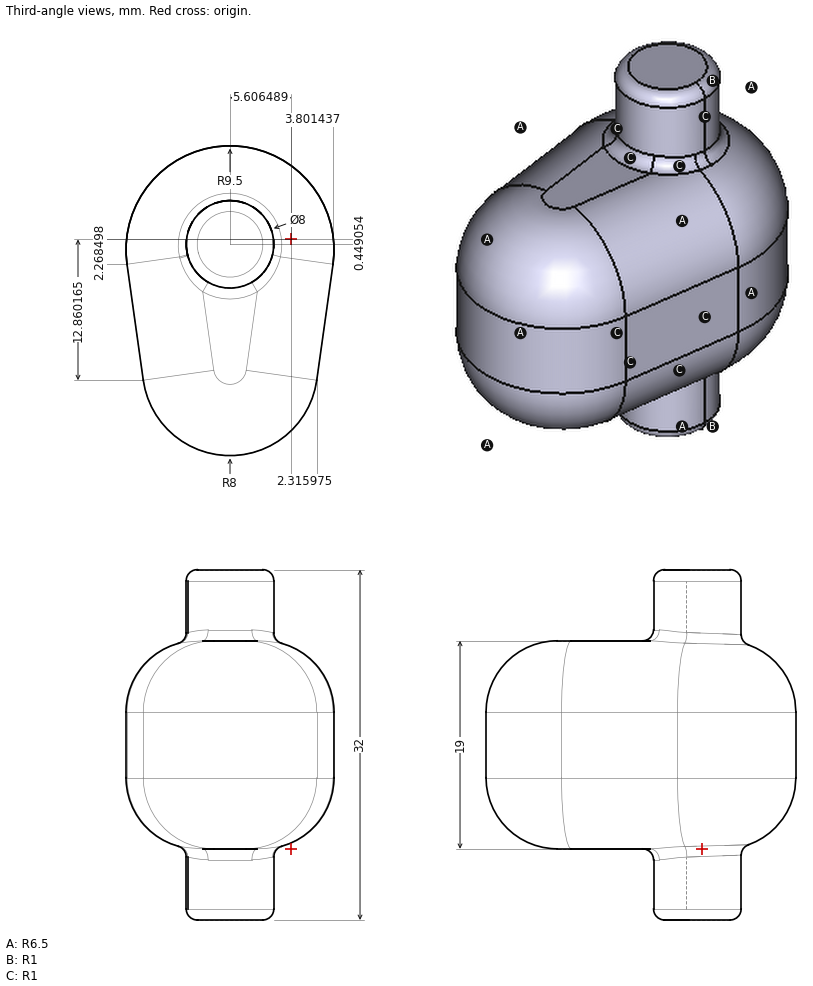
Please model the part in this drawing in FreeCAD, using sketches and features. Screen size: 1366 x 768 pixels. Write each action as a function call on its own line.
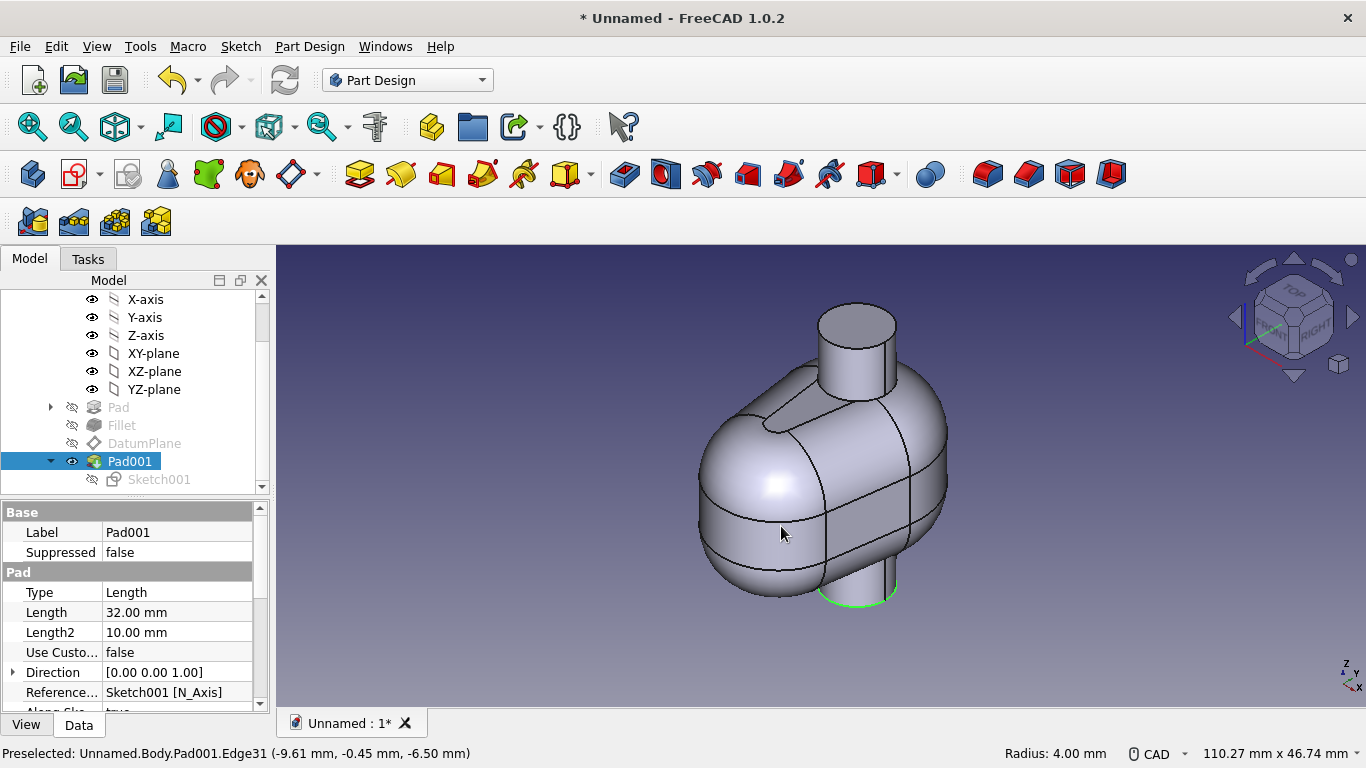
click(818, 321, ctrl)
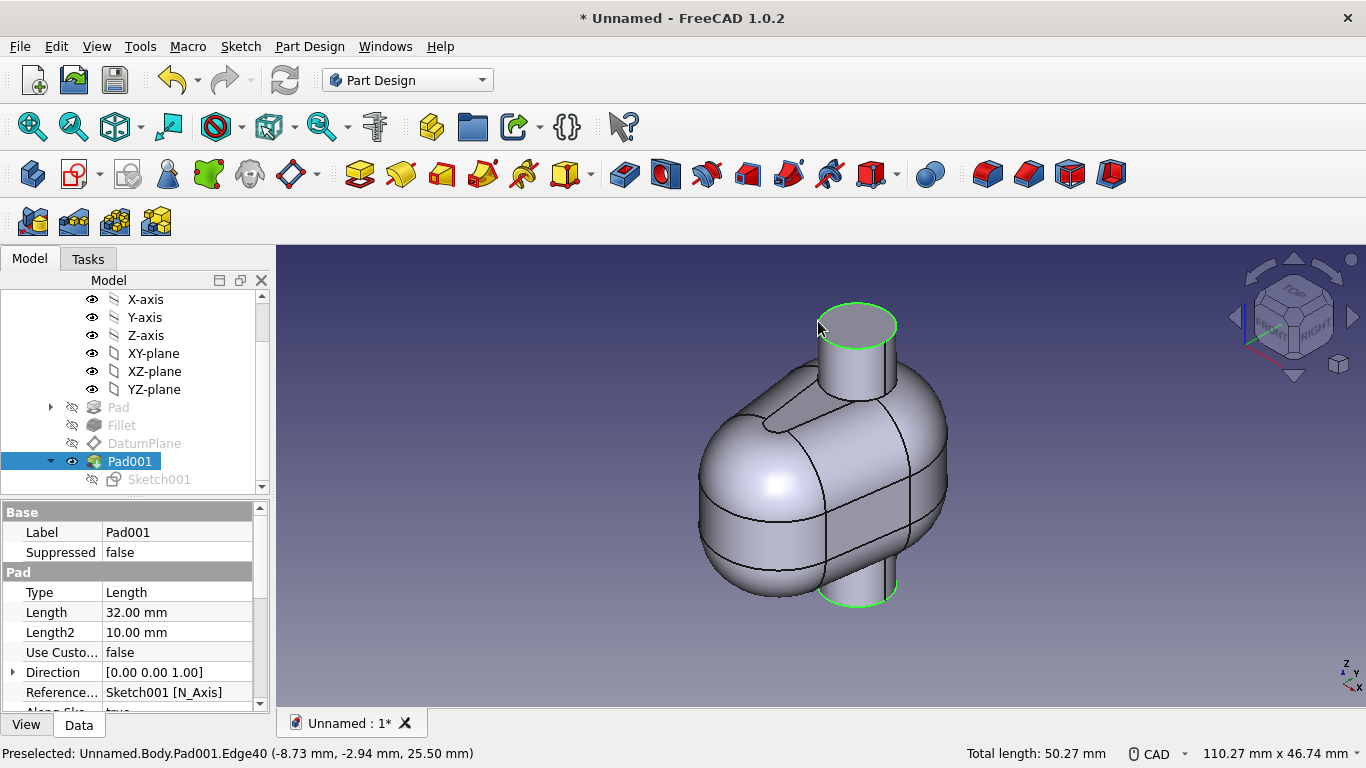
click(988, 174)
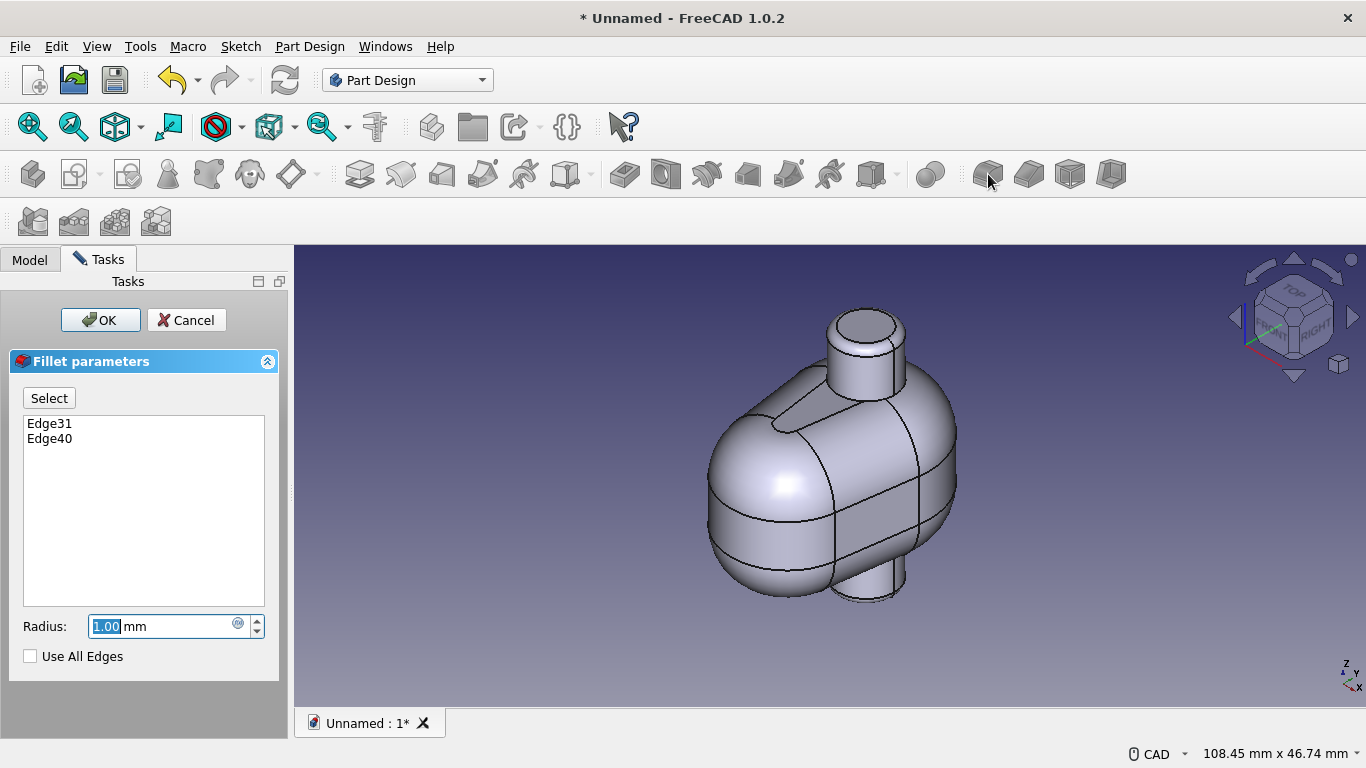
text(1)
key(Tab)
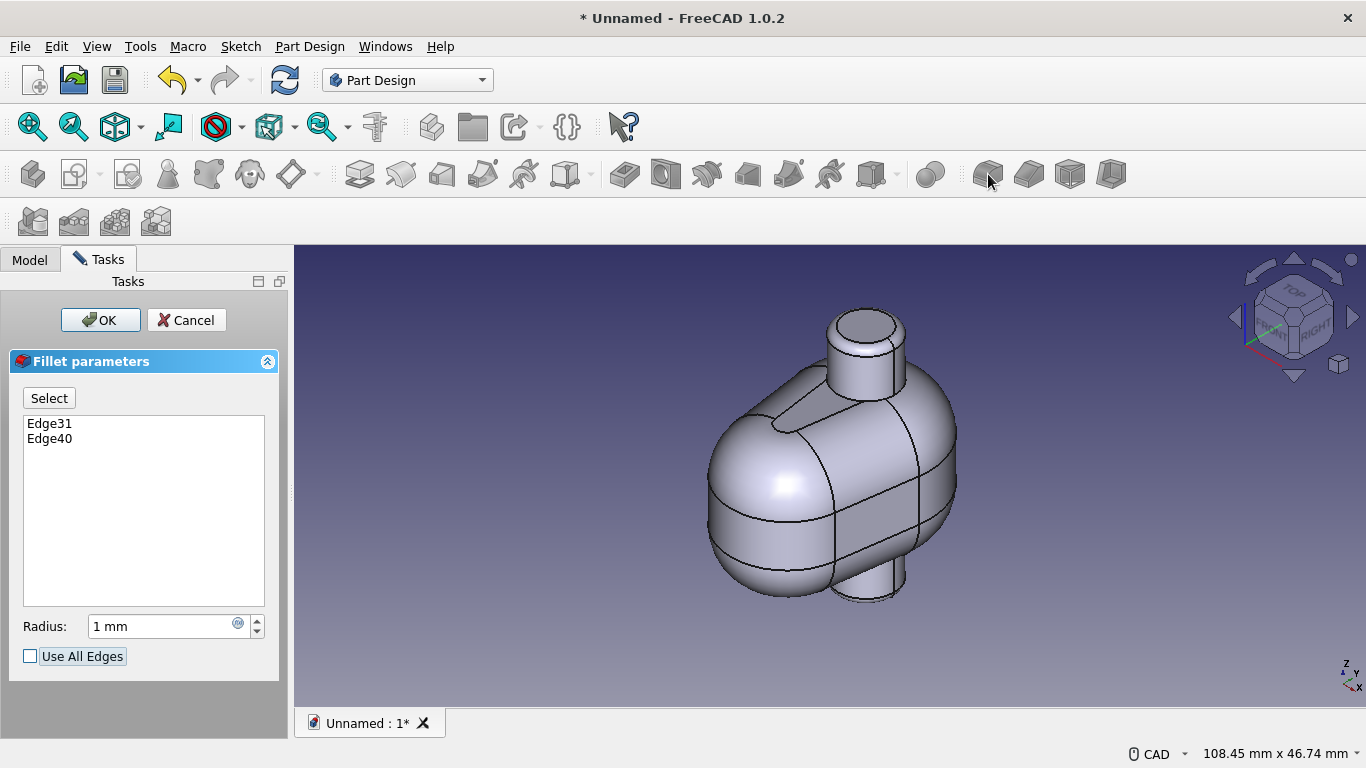
click(101, 320)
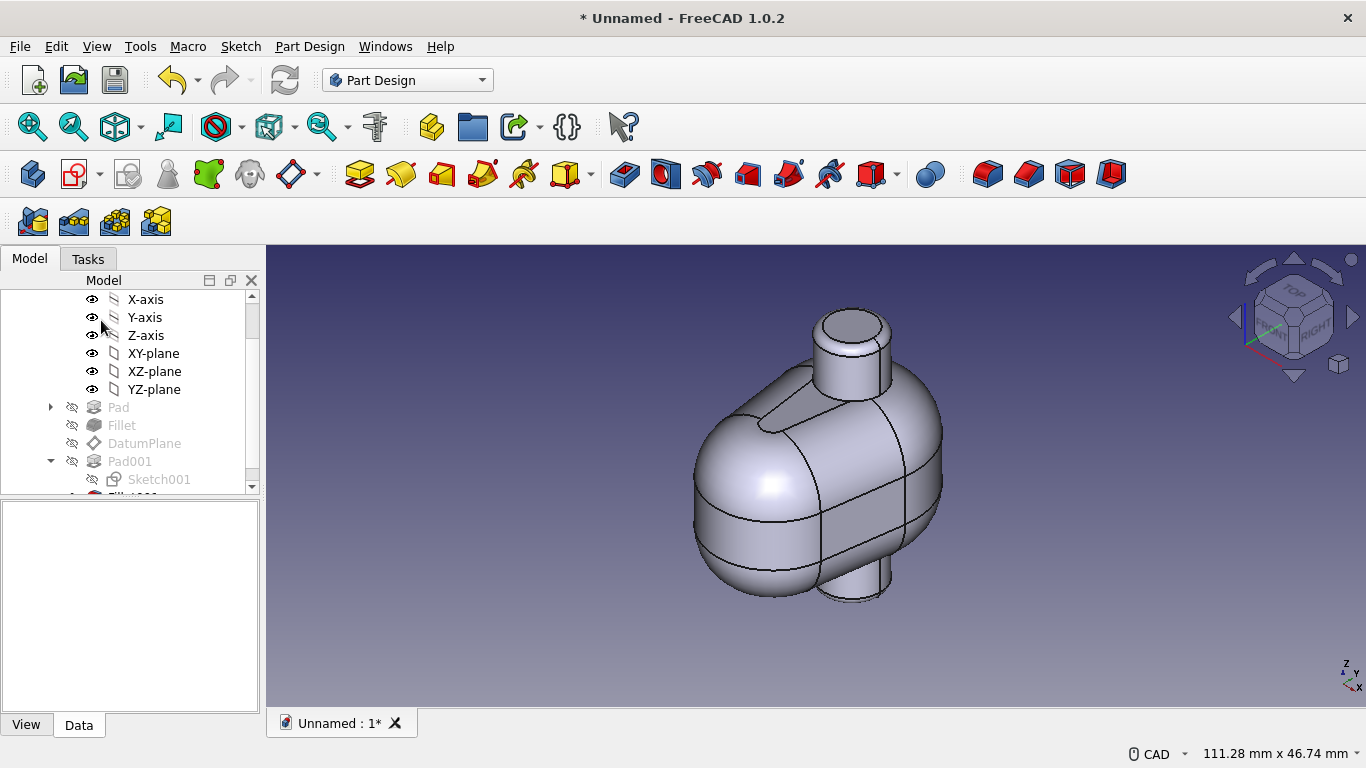
click(889, 387)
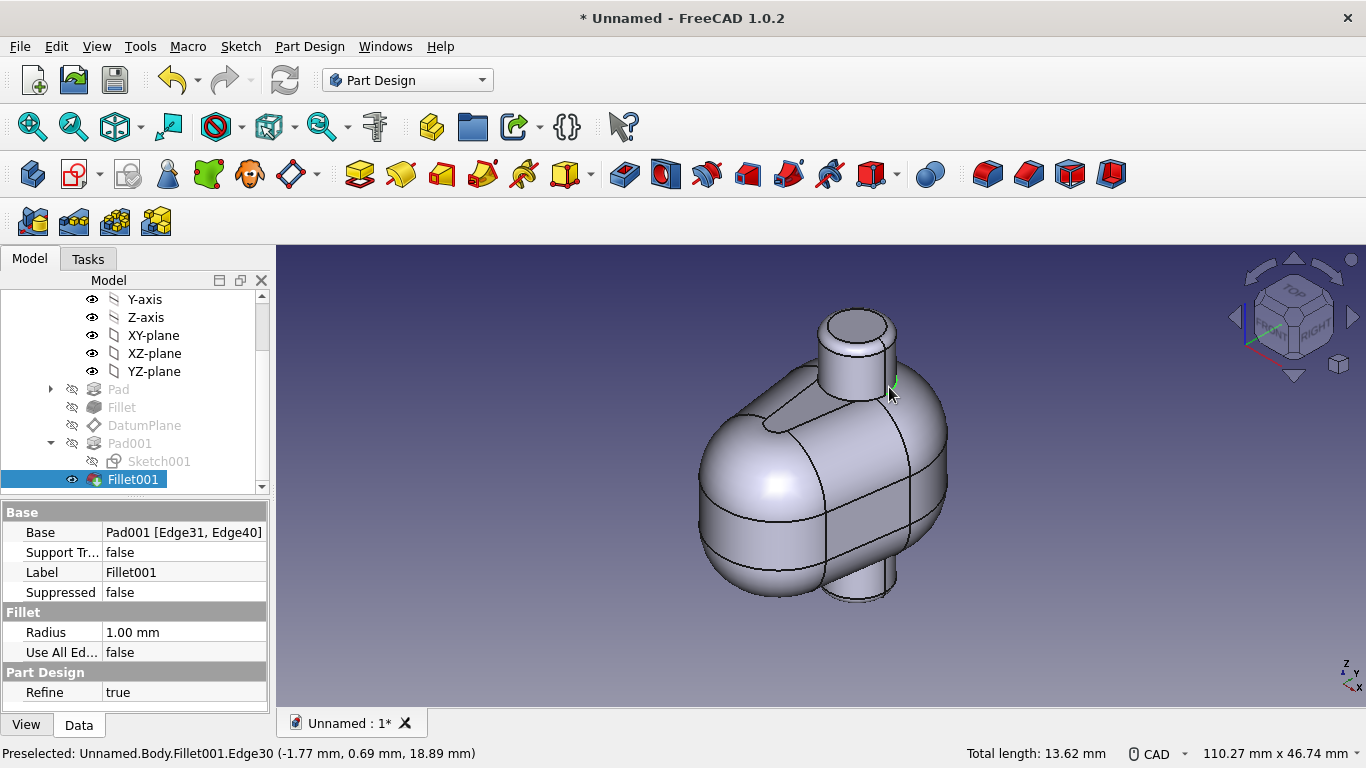
key(2)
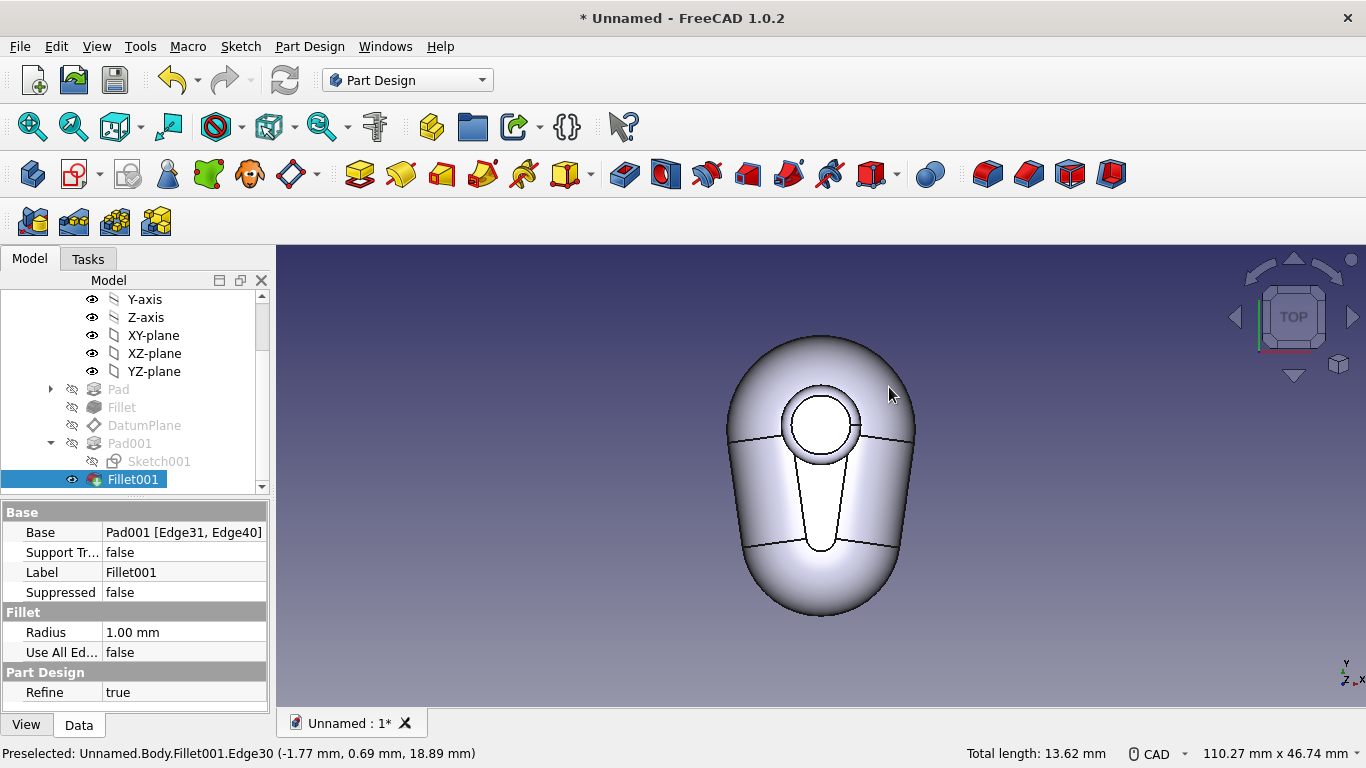
key(0)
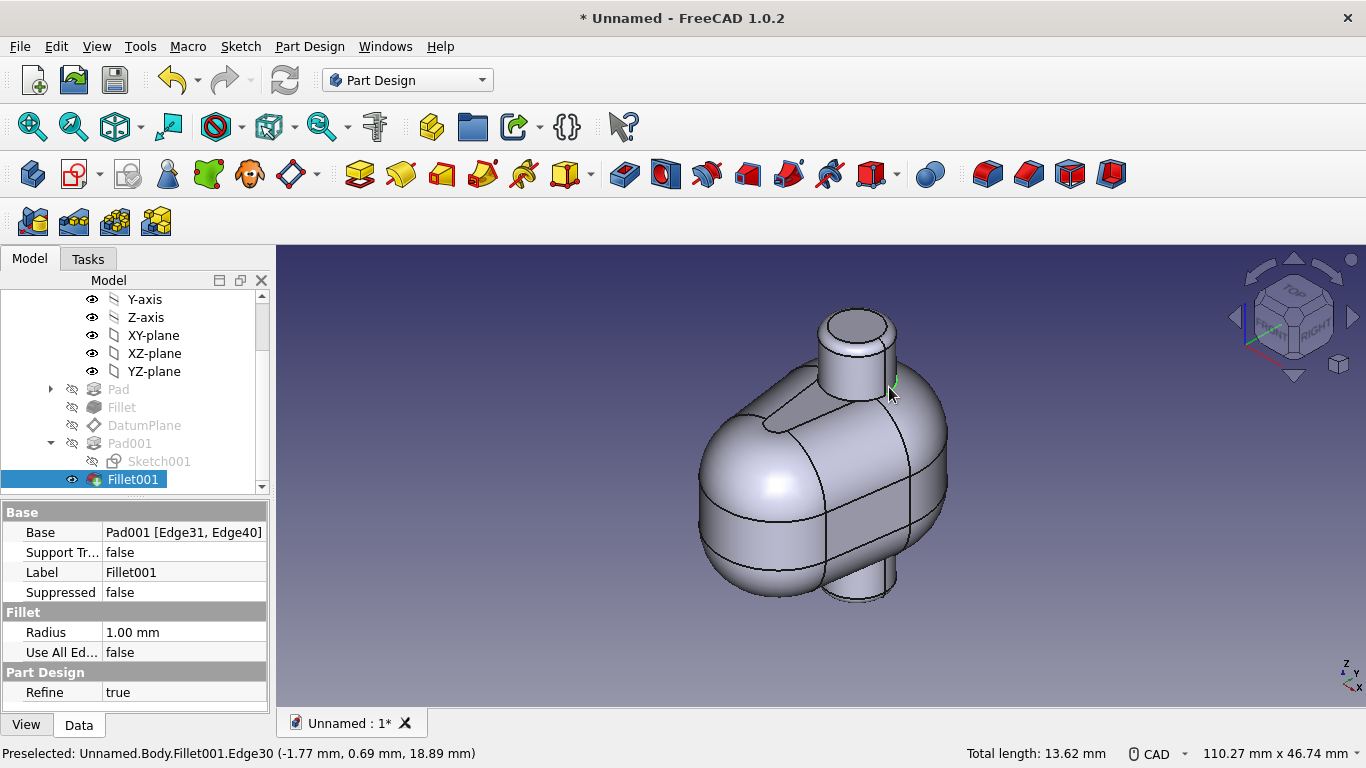
key(1)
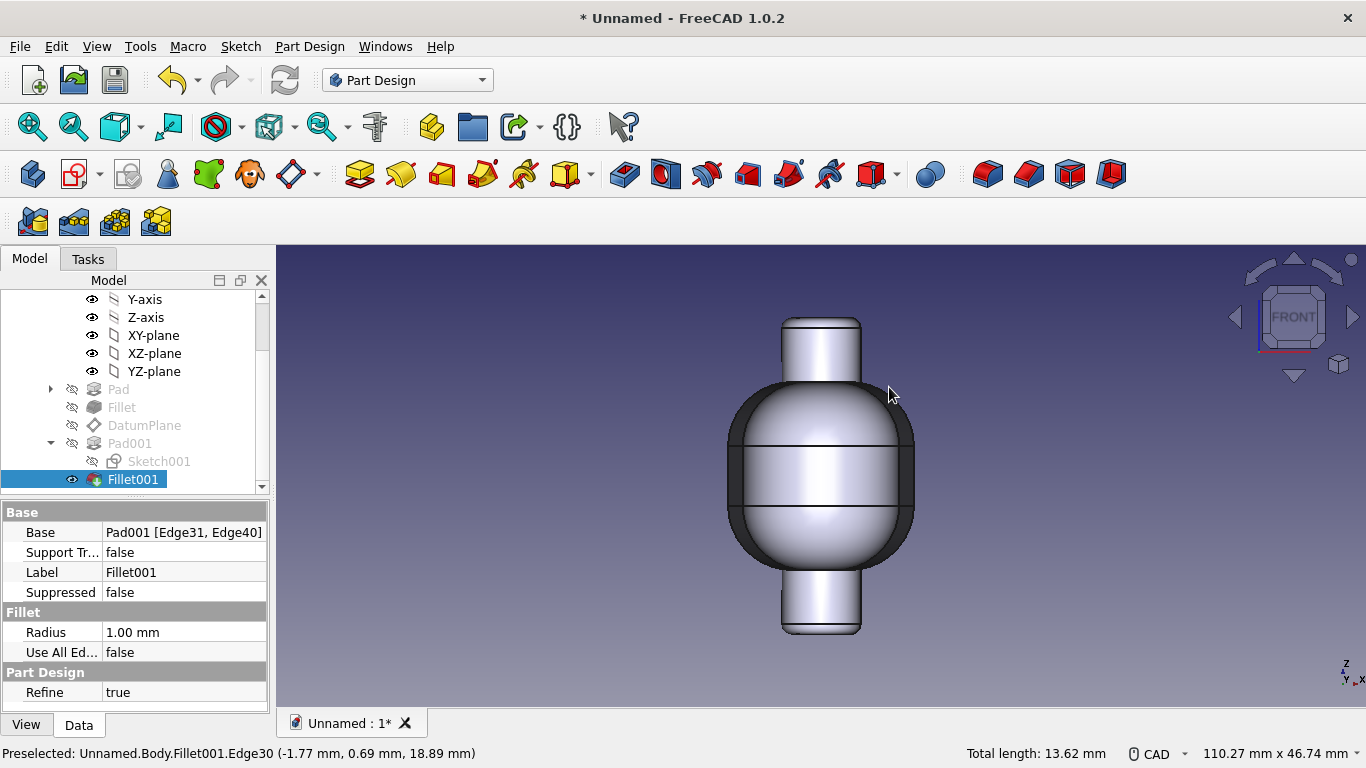
key(3)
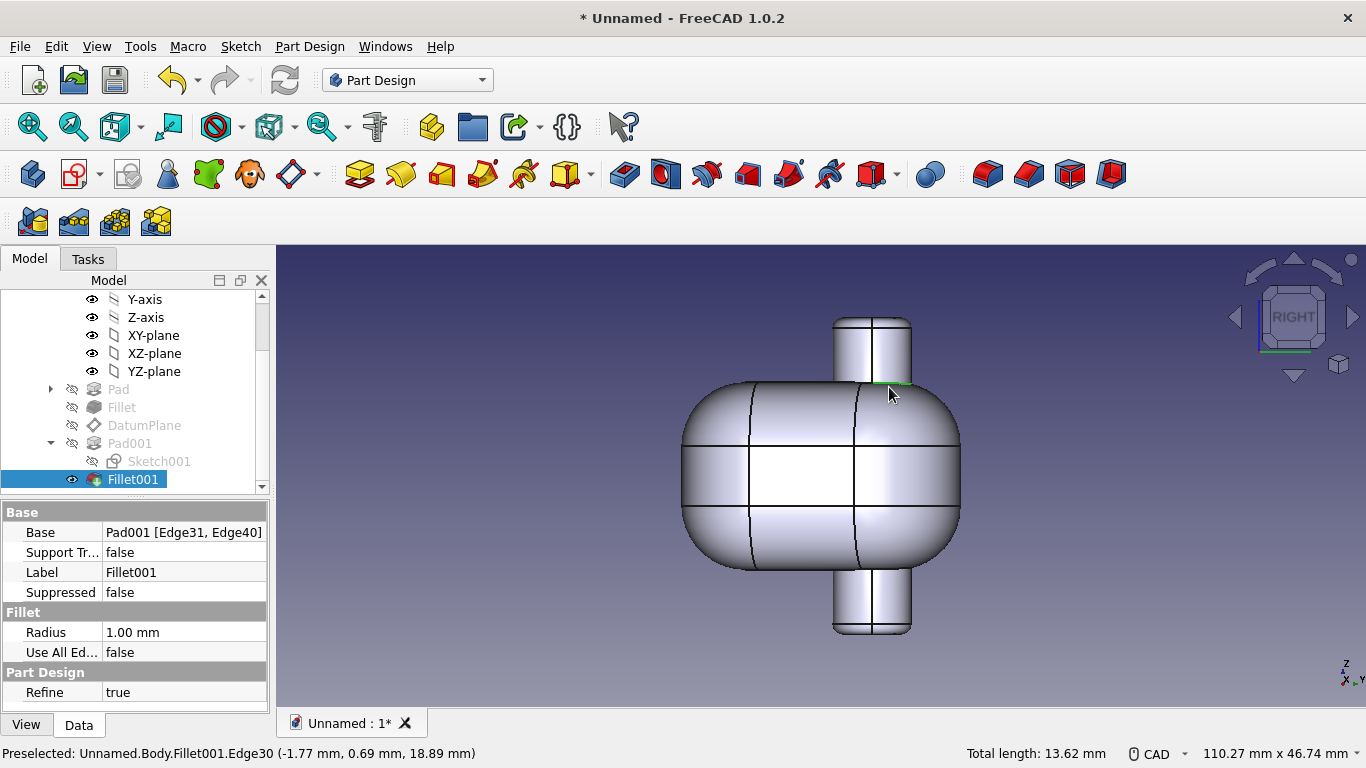
key(5)